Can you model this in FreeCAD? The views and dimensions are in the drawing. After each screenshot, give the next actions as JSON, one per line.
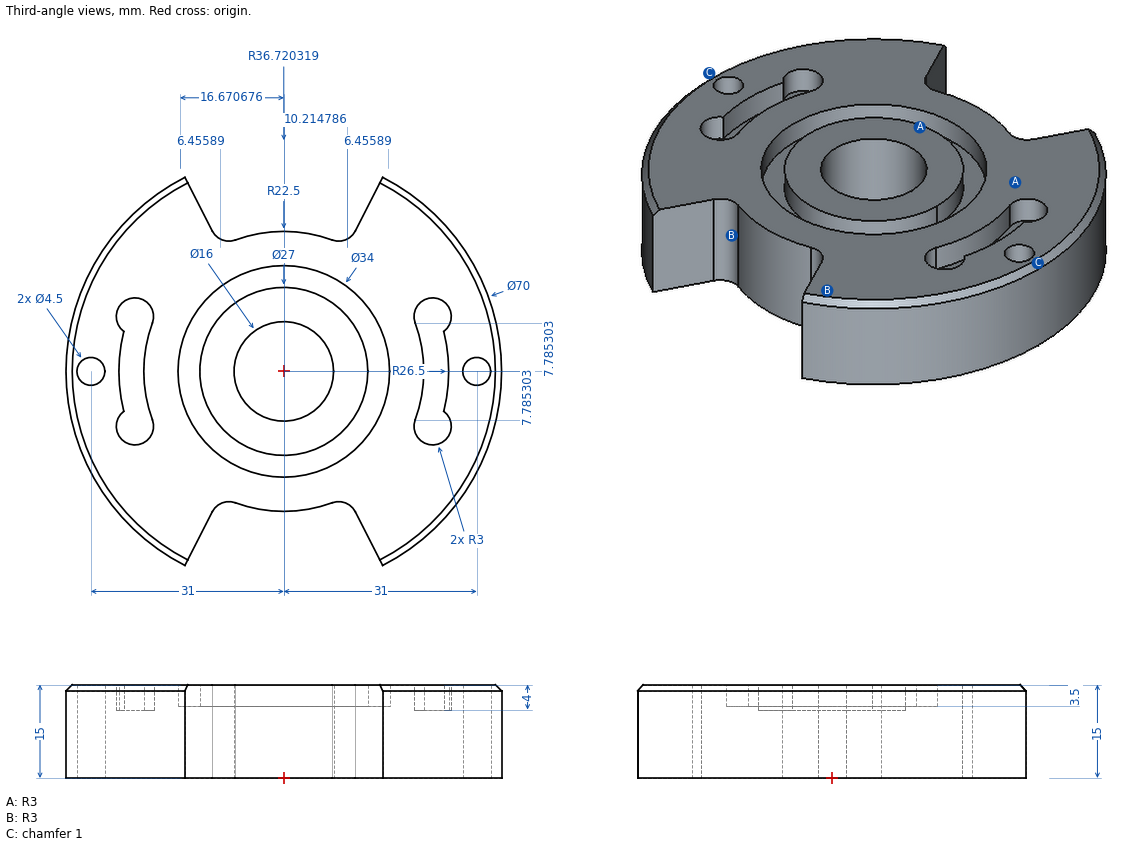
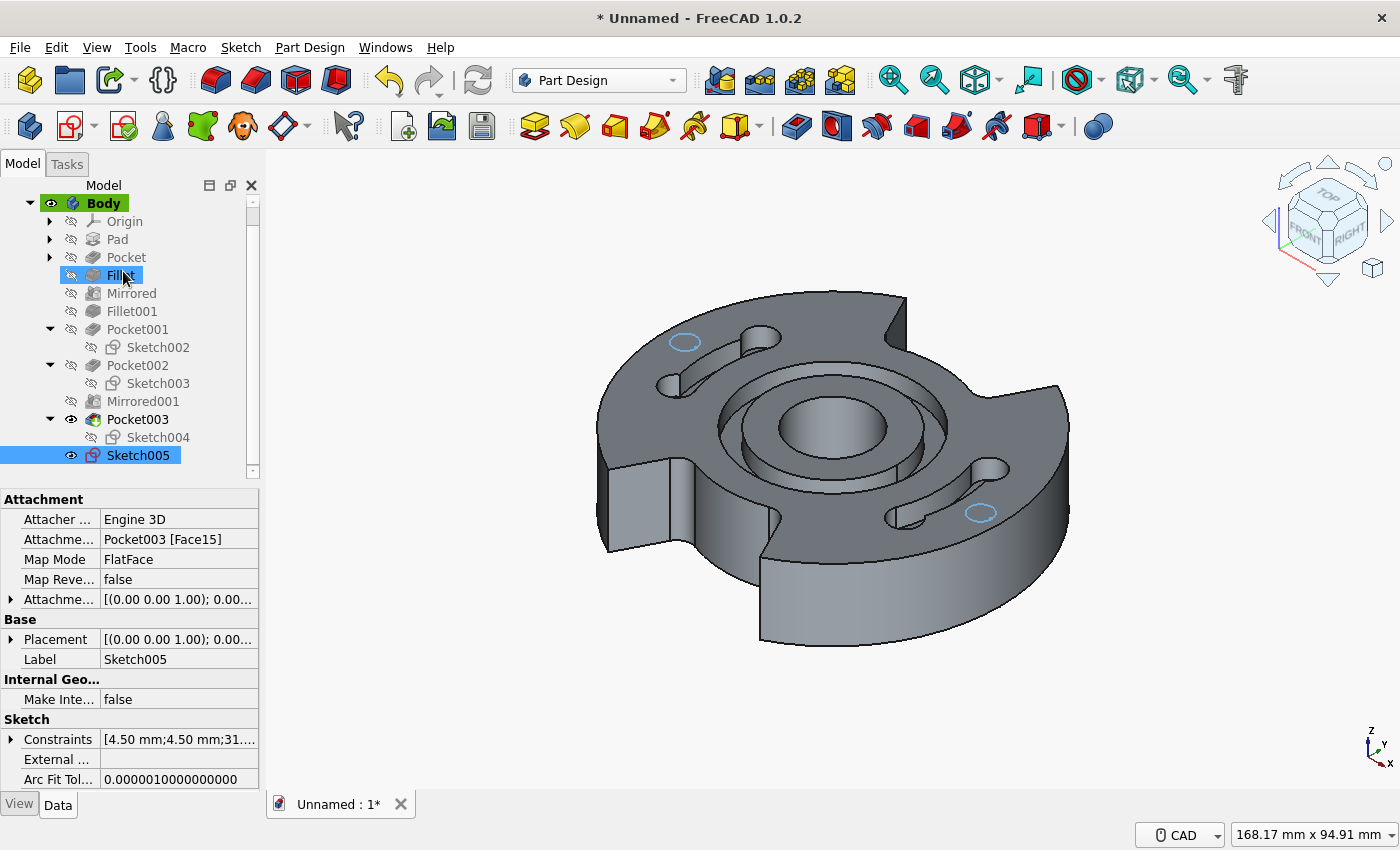
{"action": "left_click", "coordinate": [798, 126]}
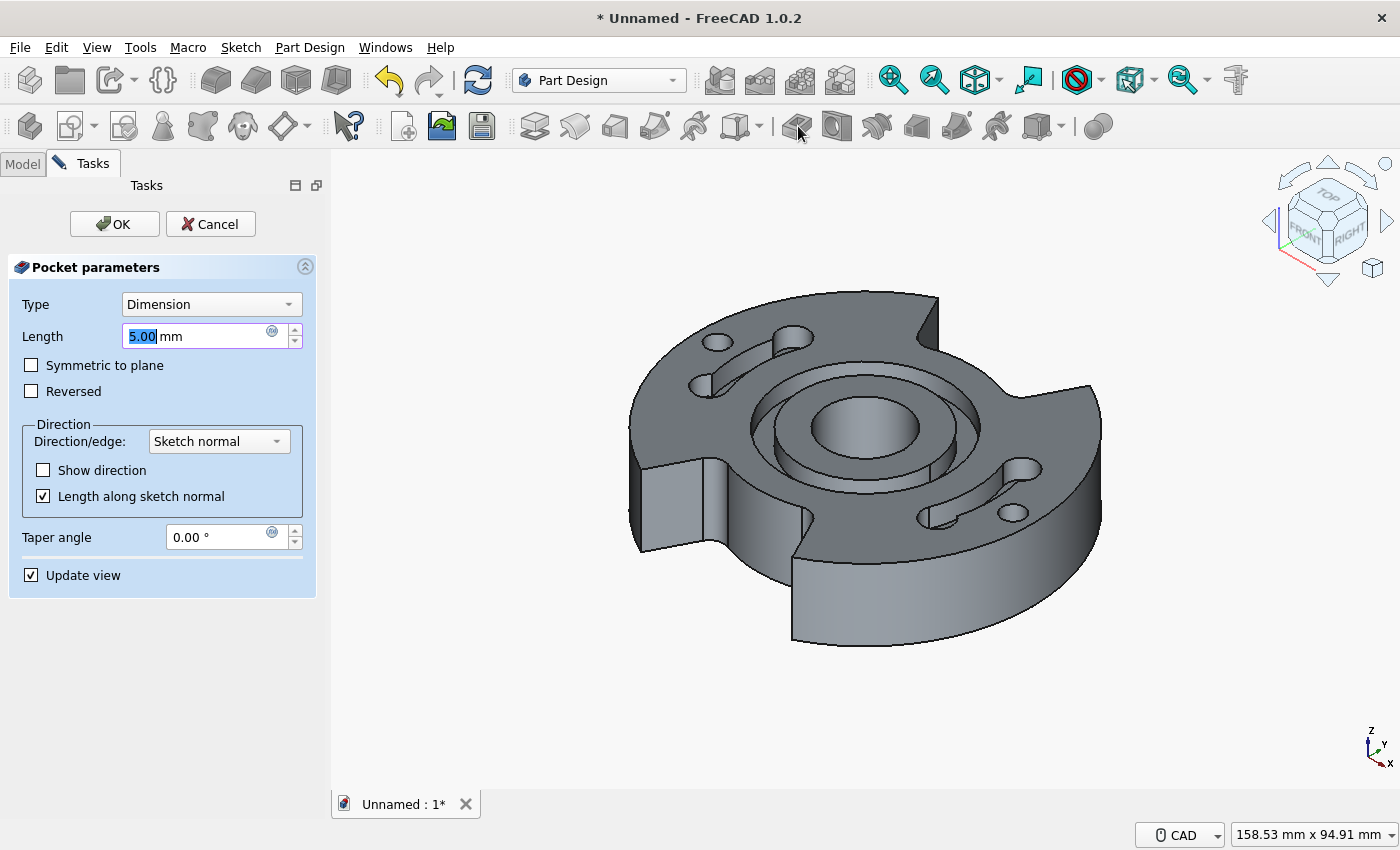
{"action": "left_click", "coordinate": [212, 304]}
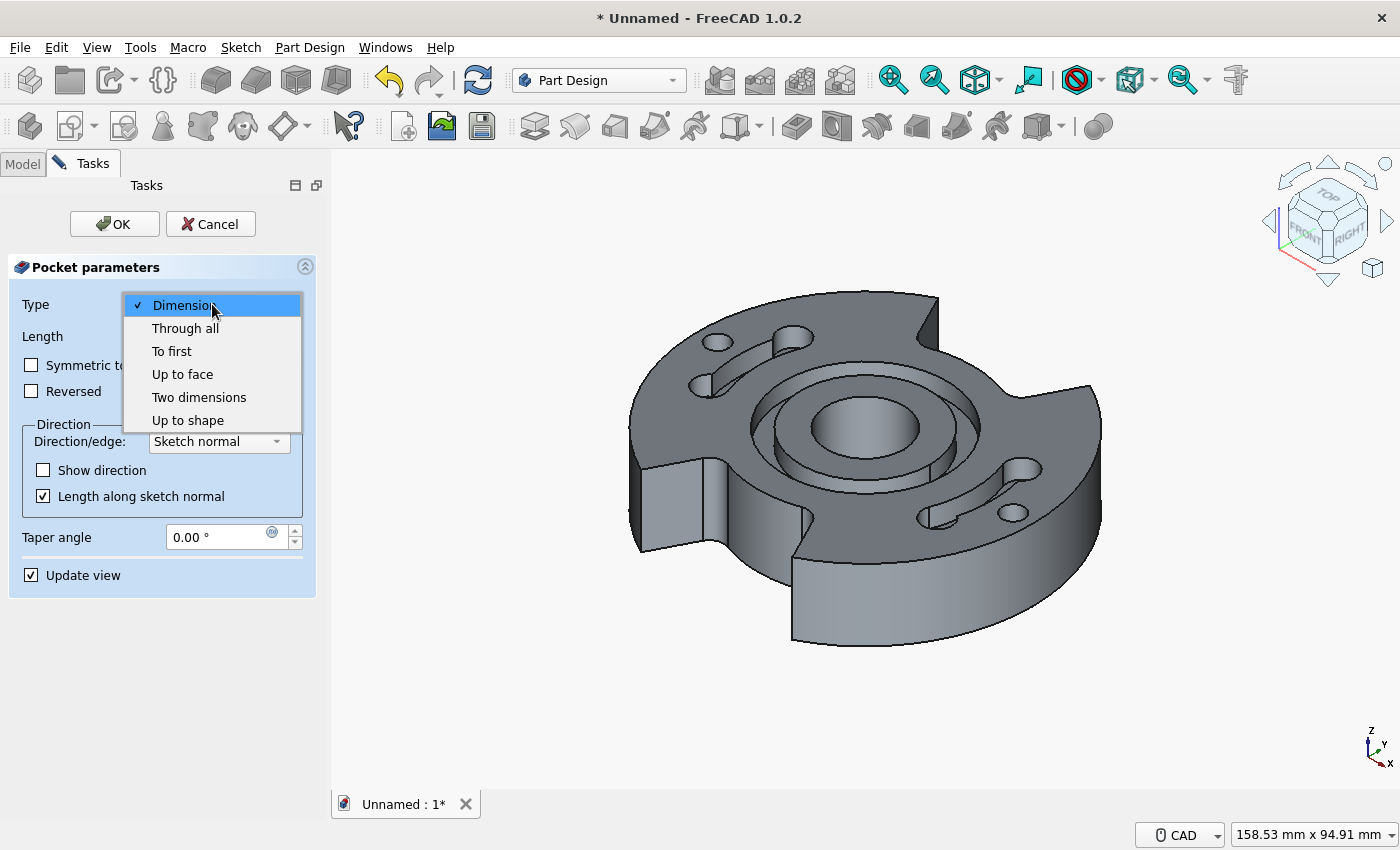
{"action": "left_click", "coordinate": [212, 328]}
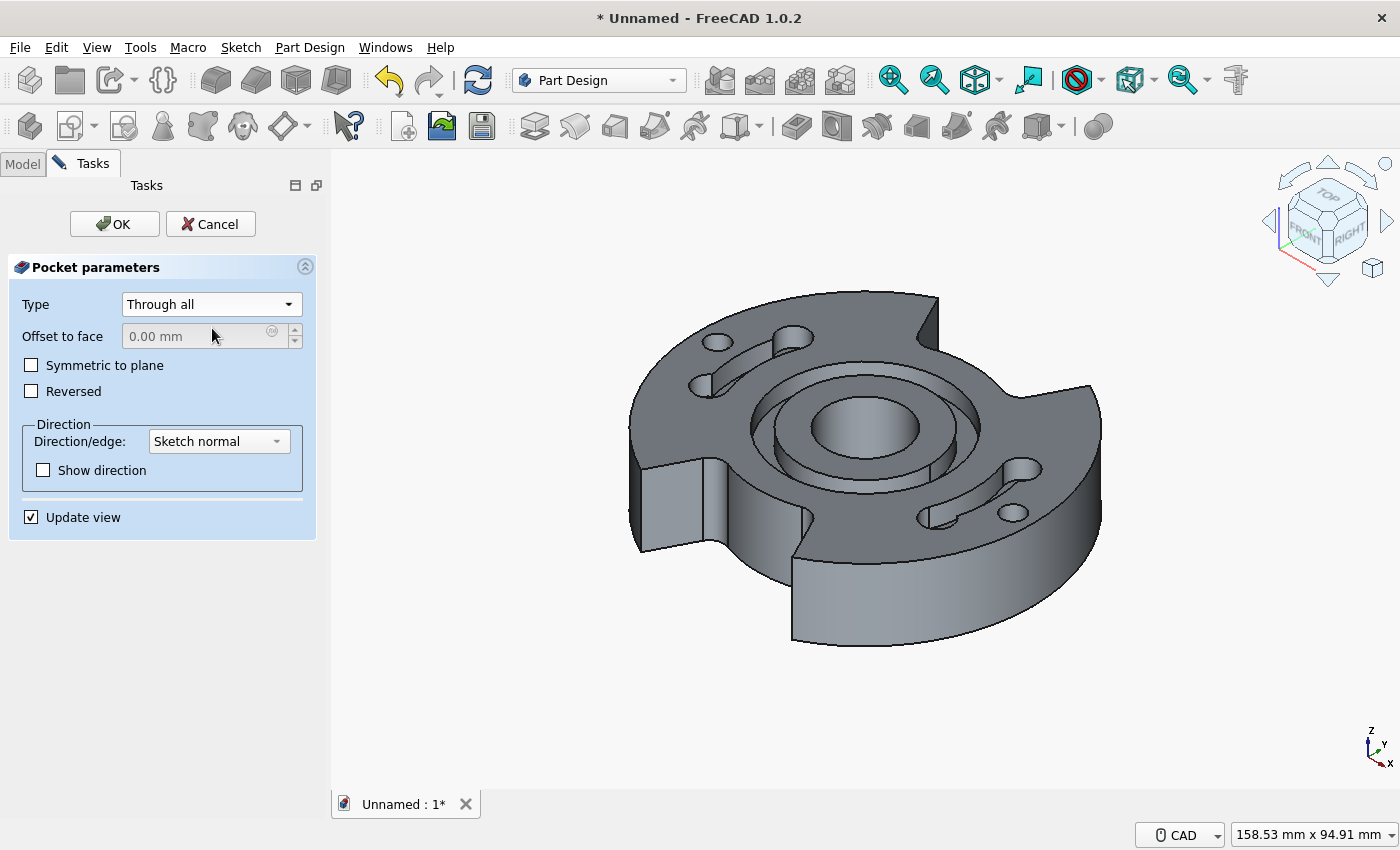
{"action": "left_click", "coordinate": [115, 224]}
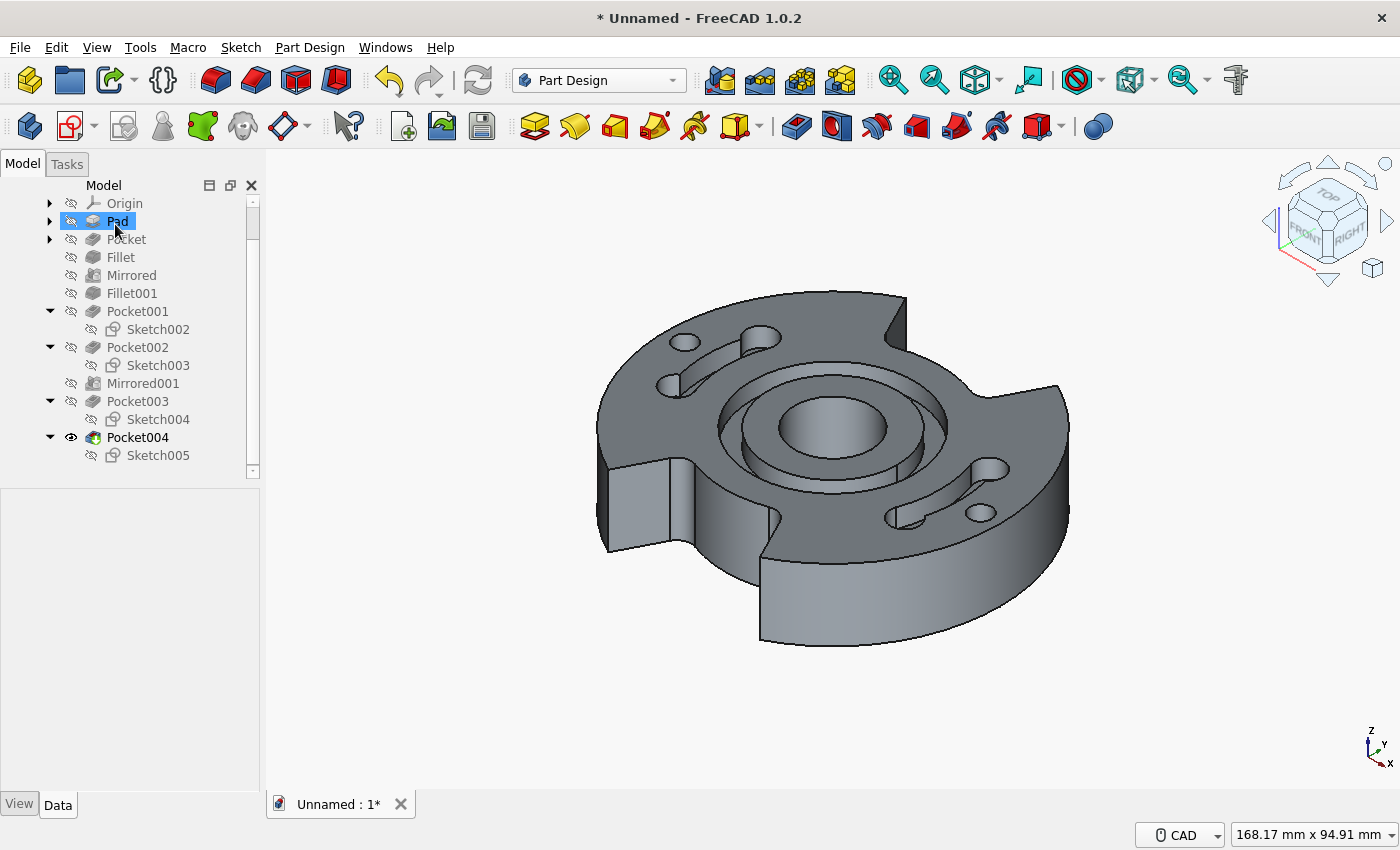
{"action": "left_click", "coordinate": [1062, 458]}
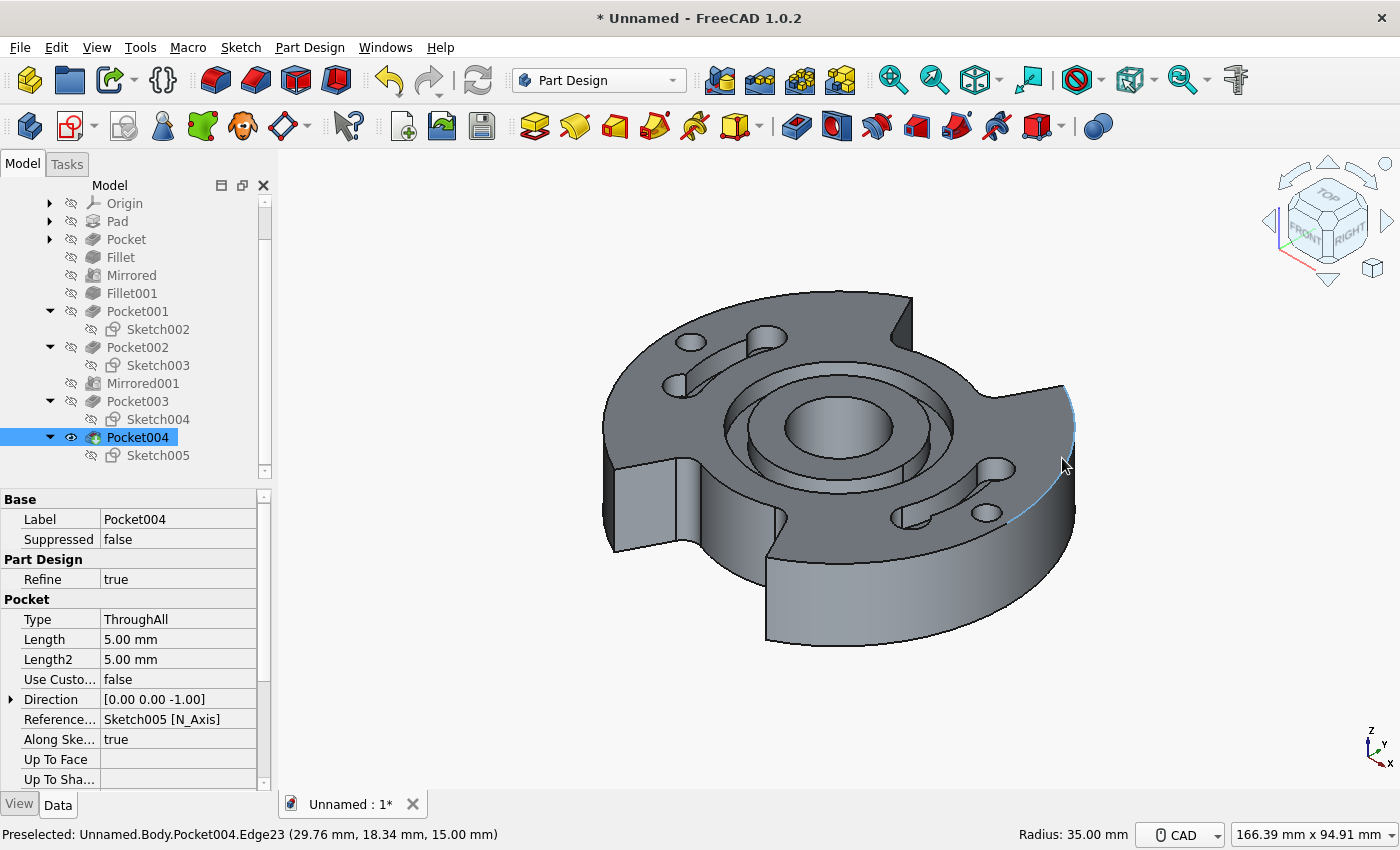
{"action": "left_click", "coordinate": [603, 433], "text": "ctrl"}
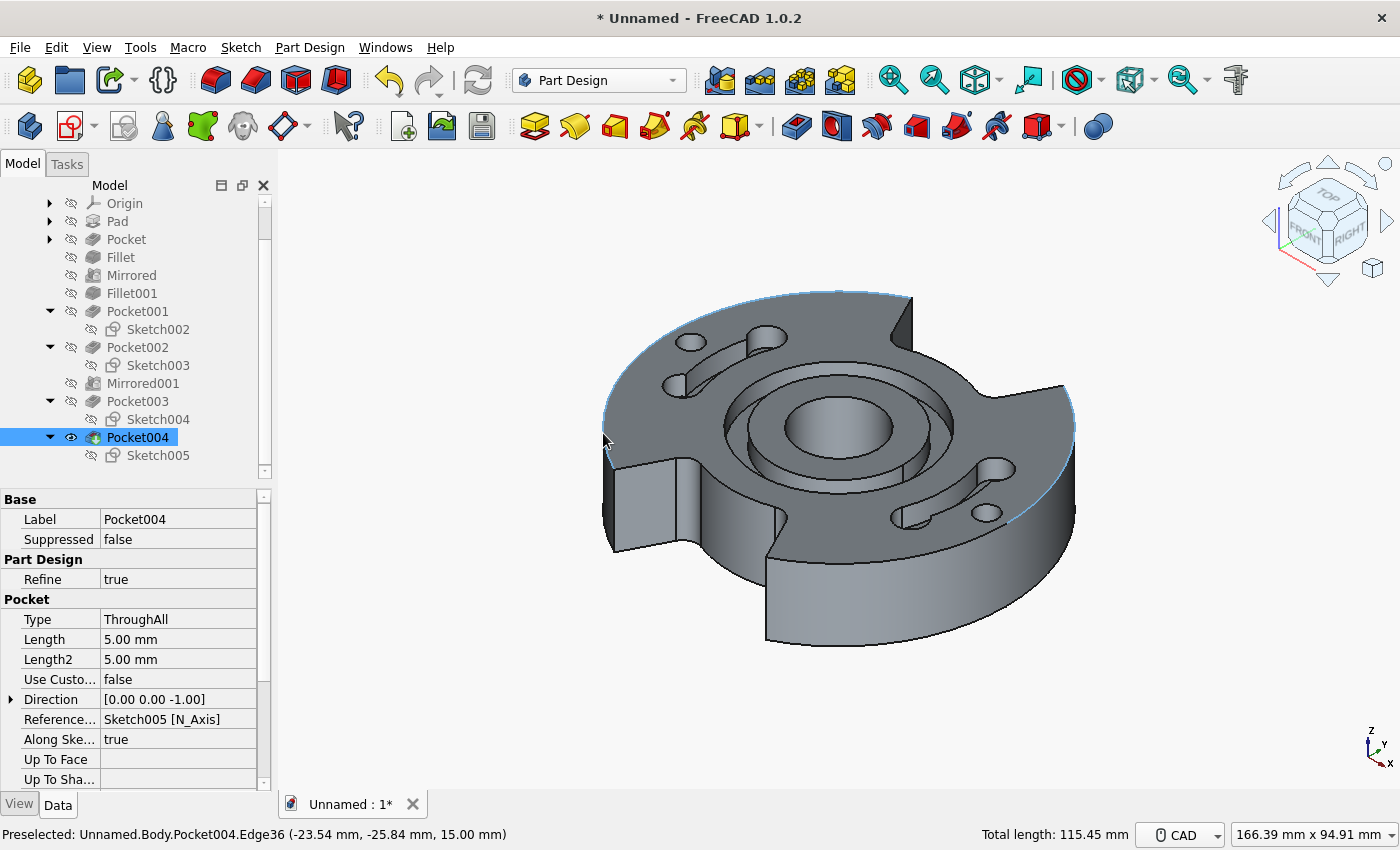
{"action": "left_click", "coordinate": [256, 80]}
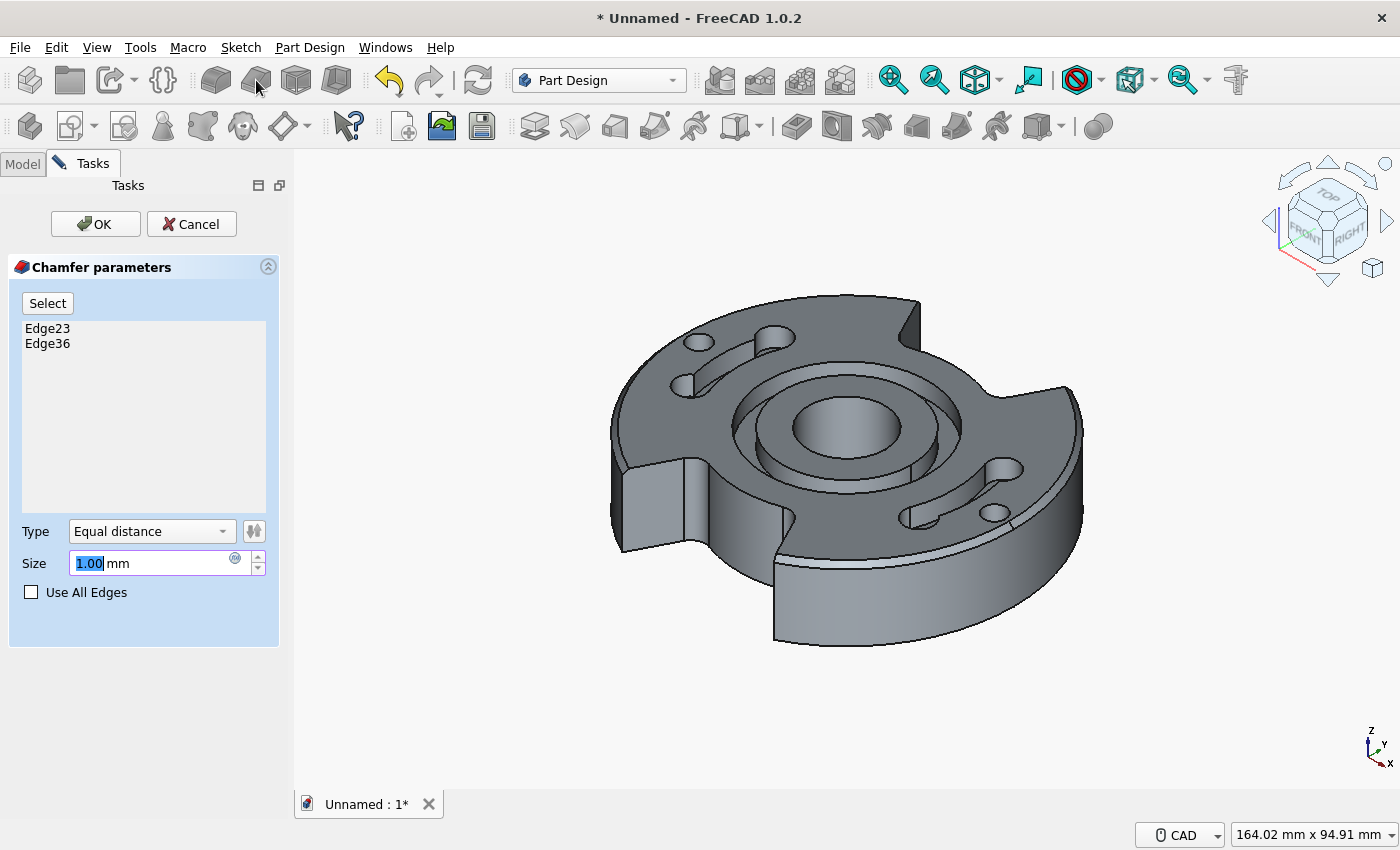
{"action": "type", "text": "1"}
{"action": "key", "text": "Tab"}